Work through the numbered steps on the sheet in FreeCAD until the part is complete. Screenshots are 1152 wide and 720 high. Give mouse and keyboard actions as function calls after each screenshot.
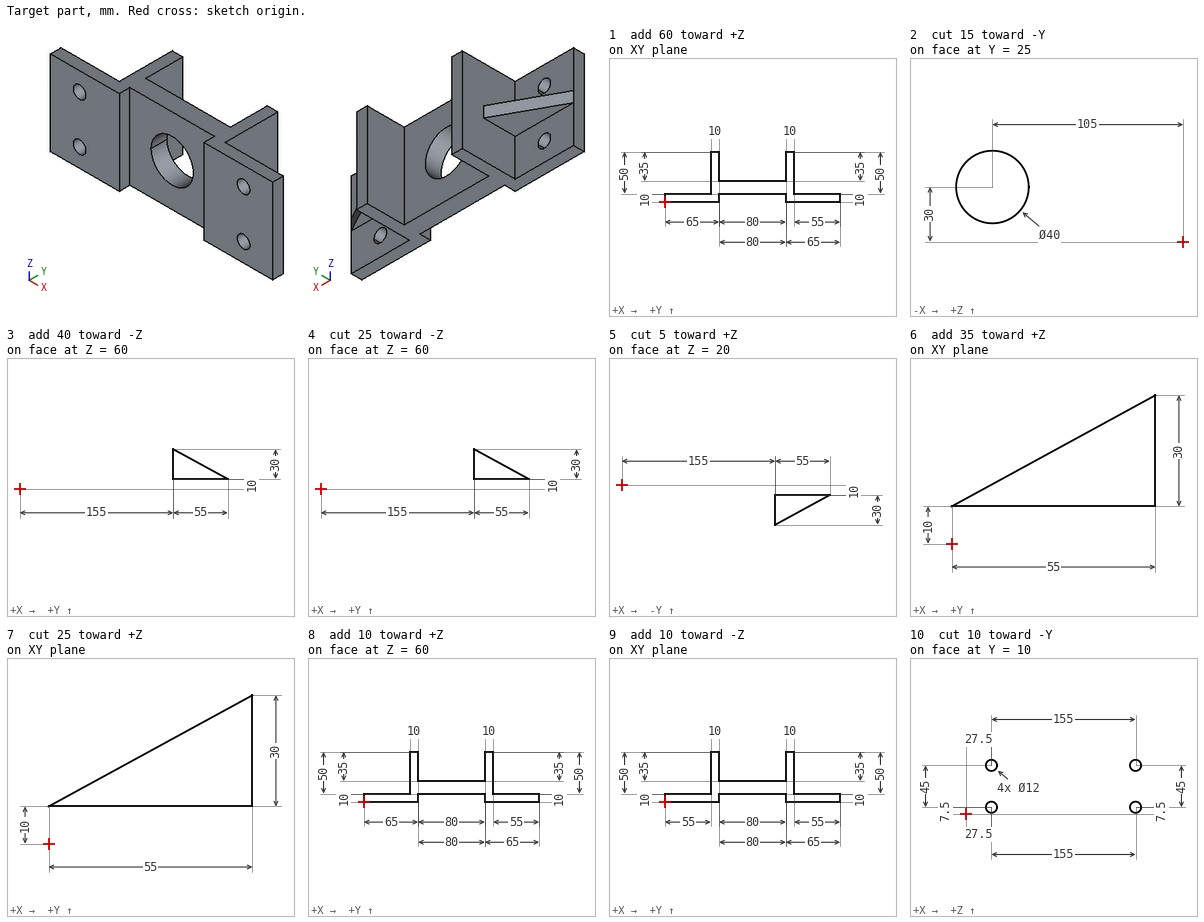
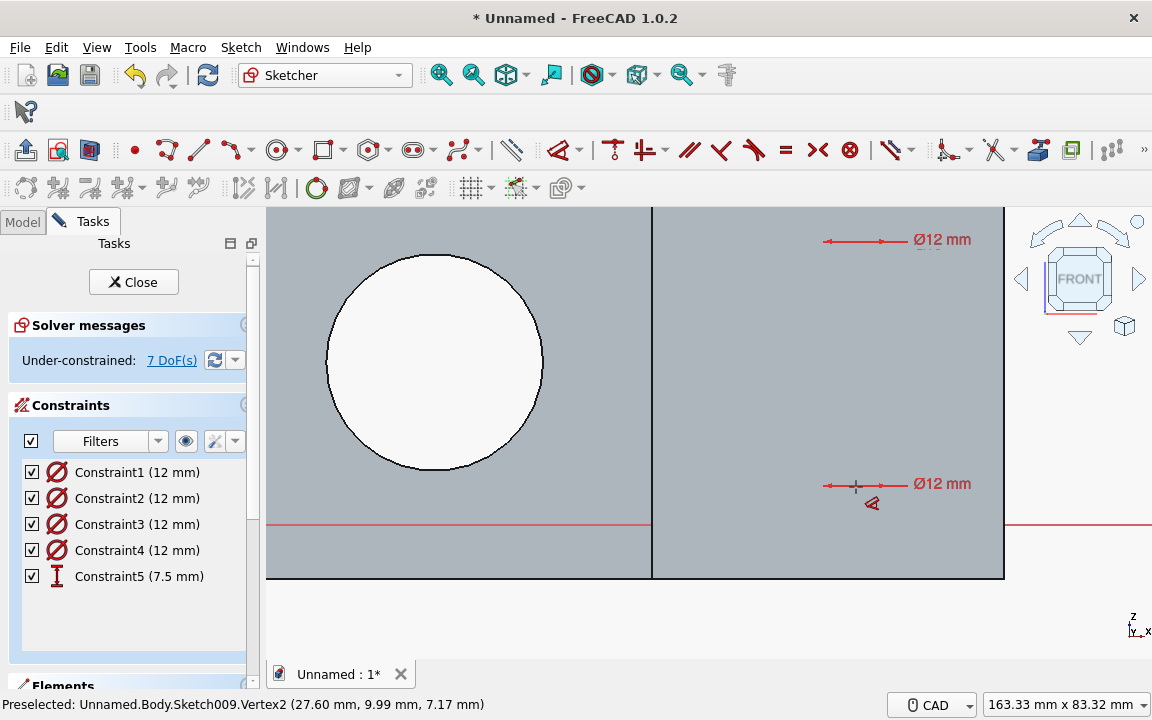
click(856, 486)
click(914, 506)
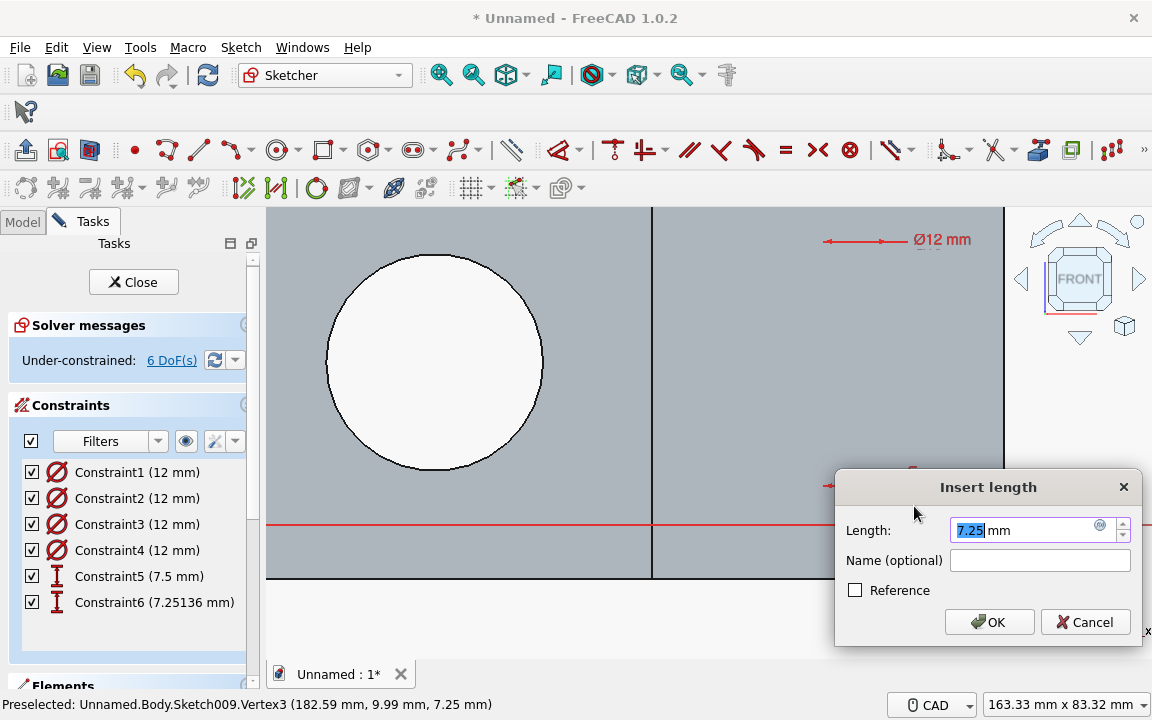
text(7.5)
key(Return)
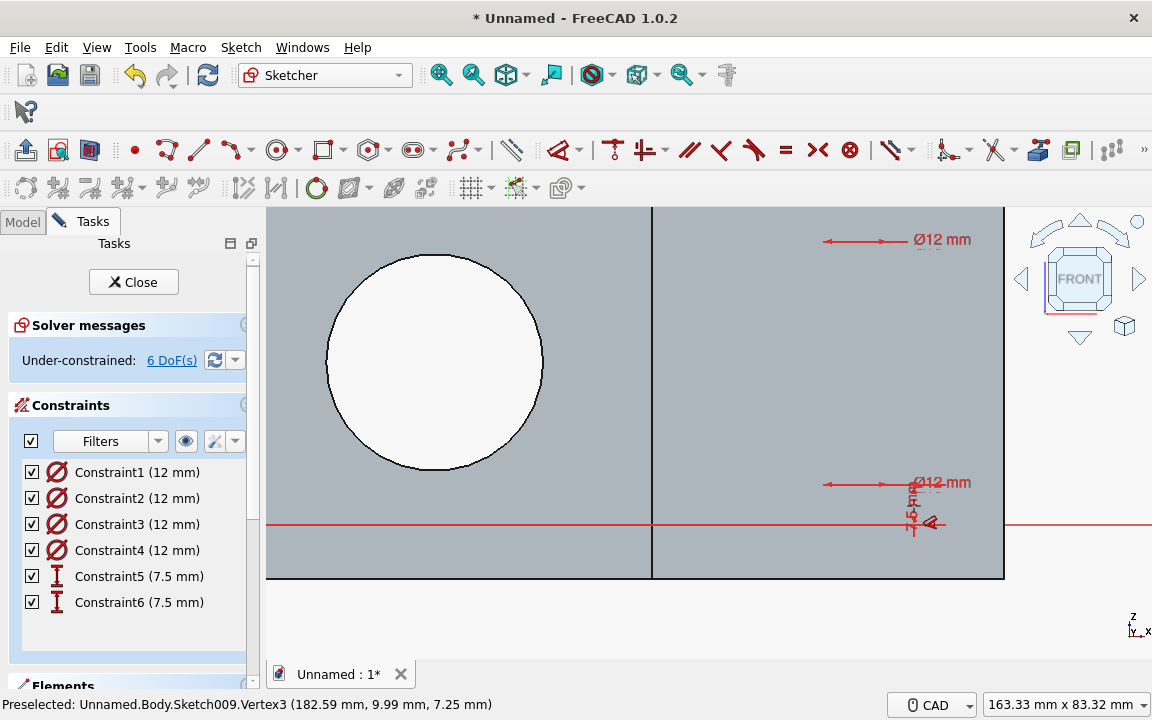
scroll(856, 487, down, 4)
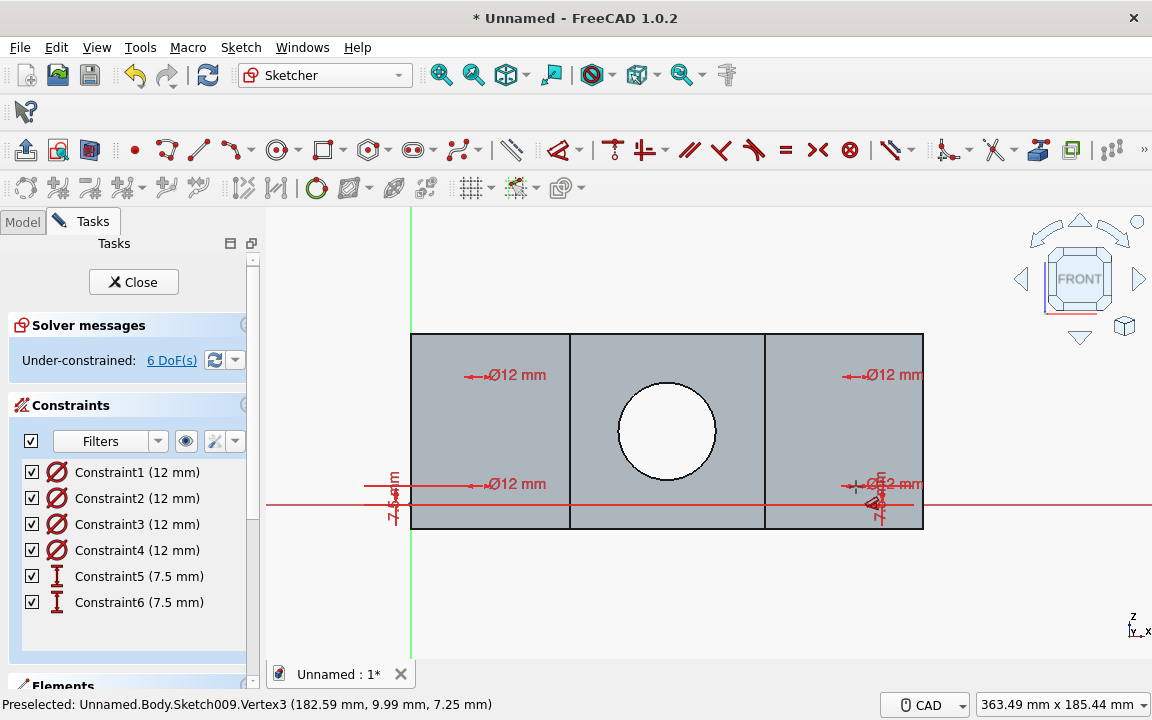
click(478, 377)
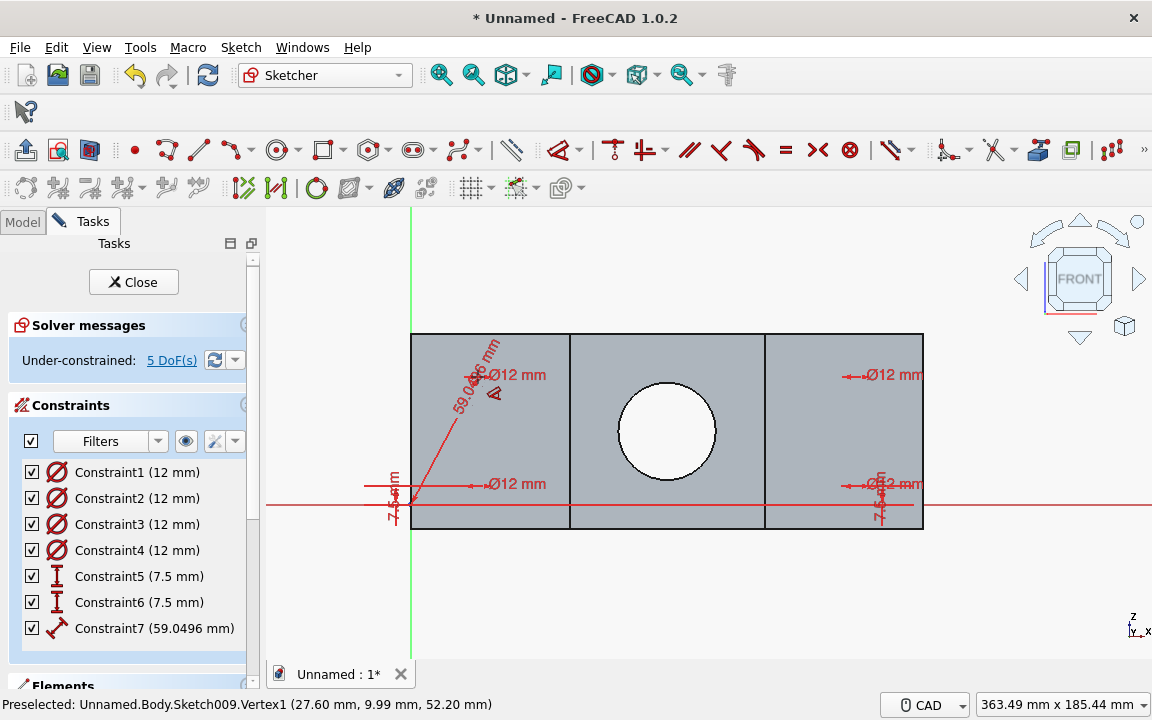
click(478, 486)
click(444, 432)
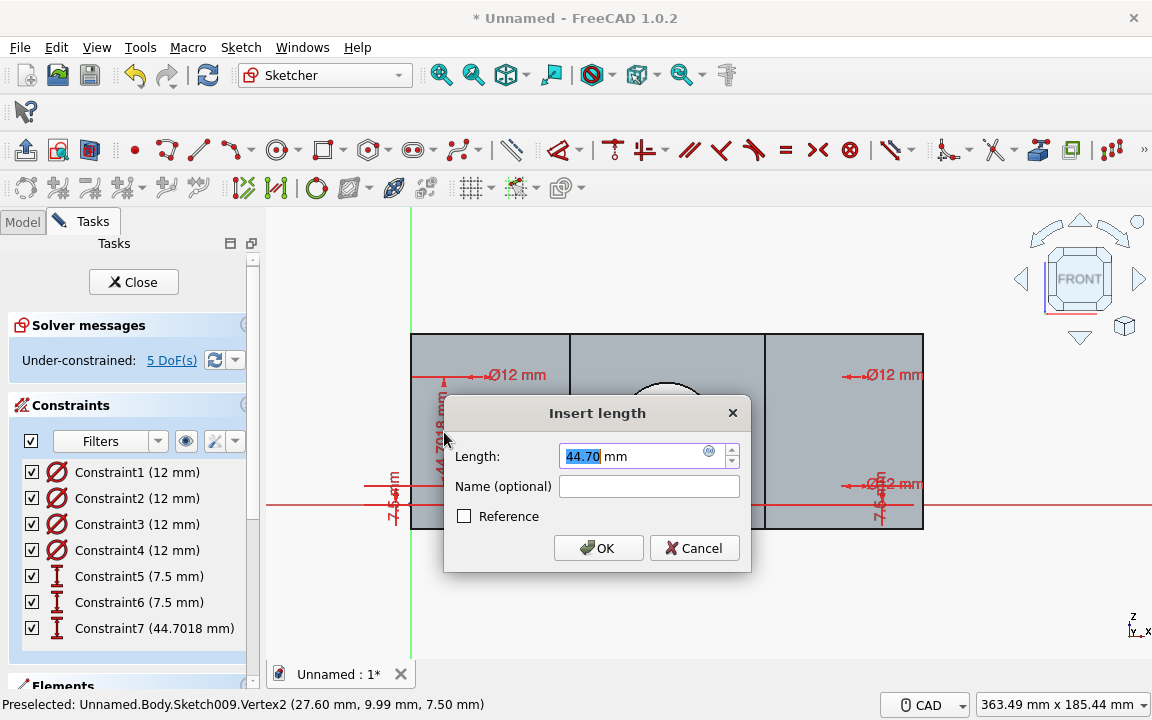
text(45)
key(Return)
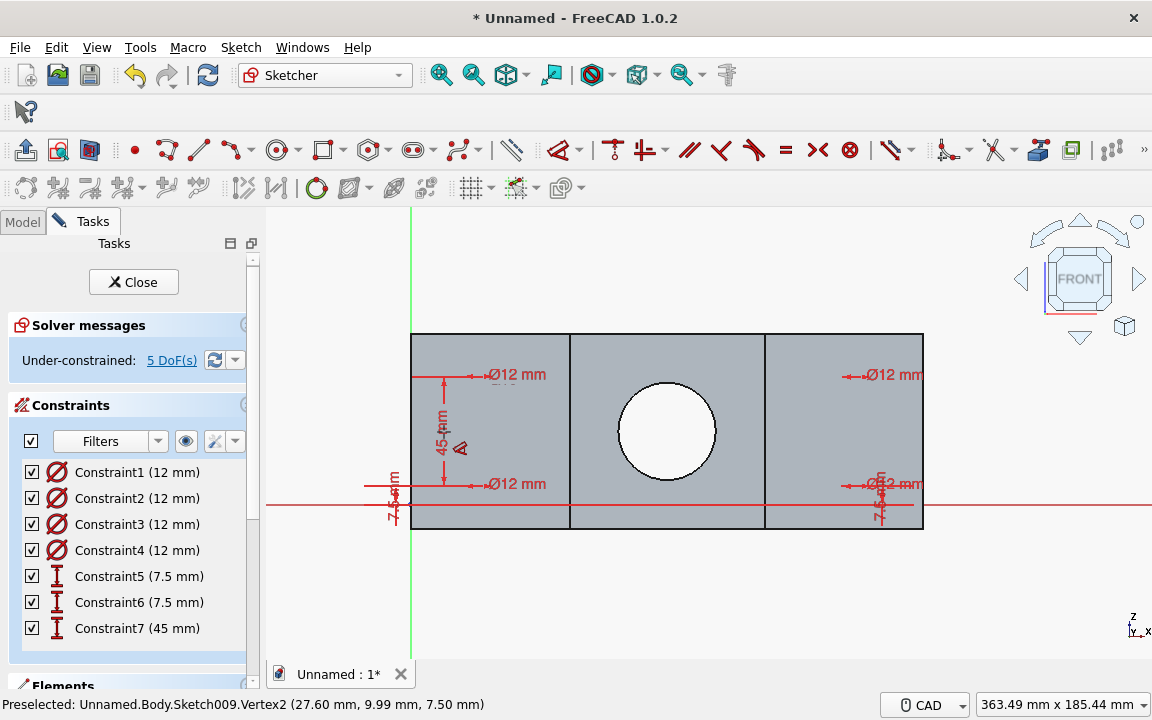
click(856, 486)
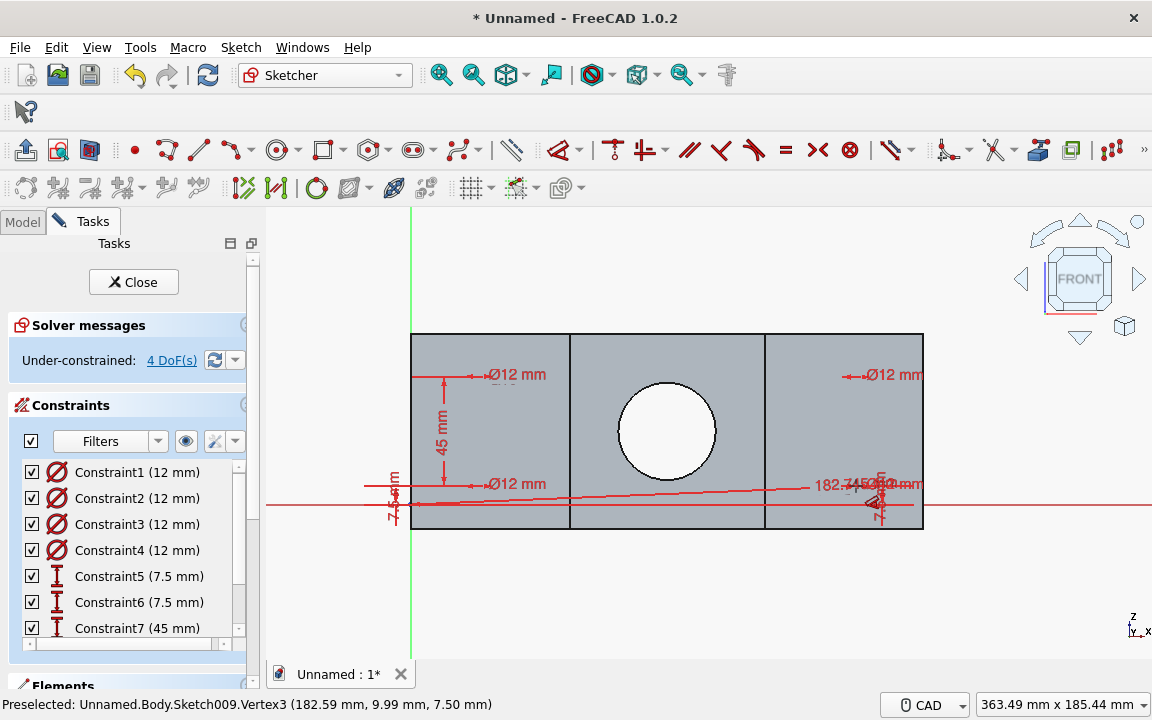
click(856, 377)
click(890, 432)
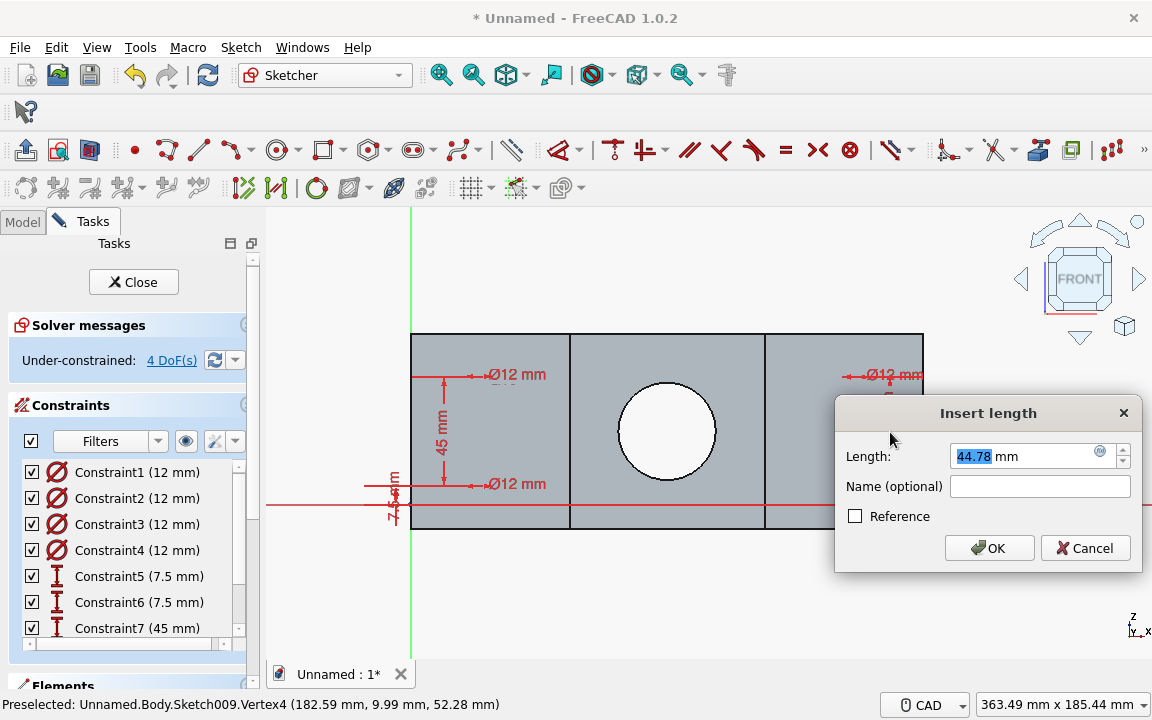
text(45)
key(Return)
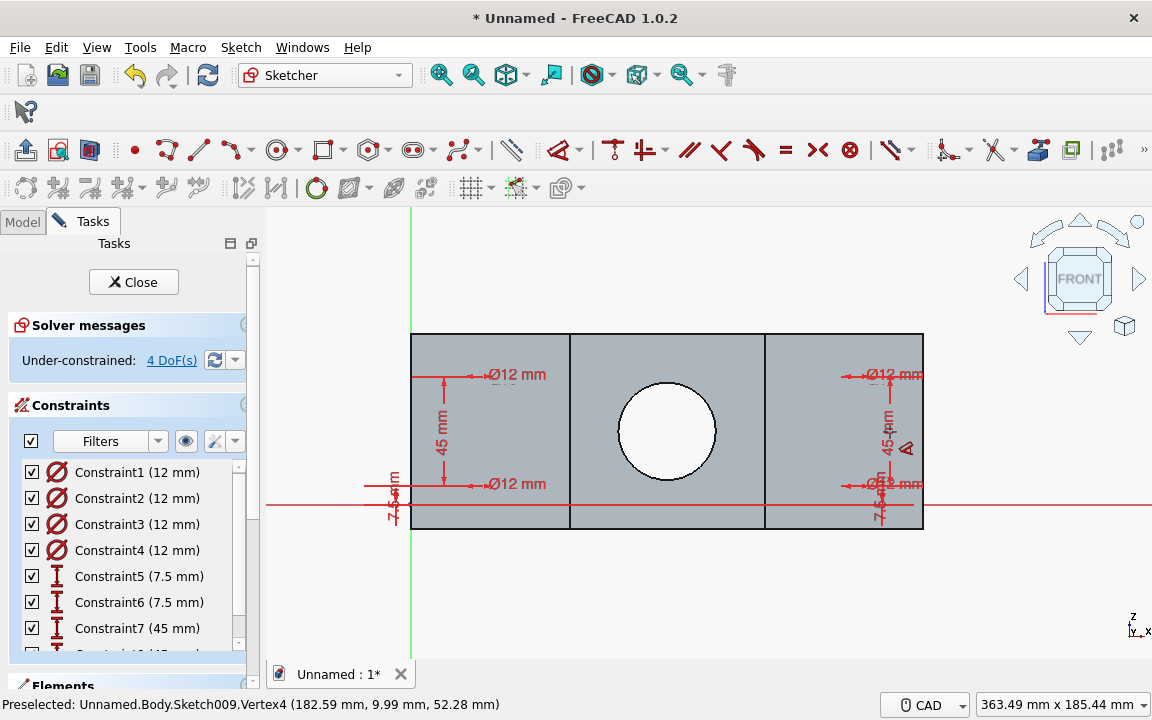
click(478, 377)
click(445, 539)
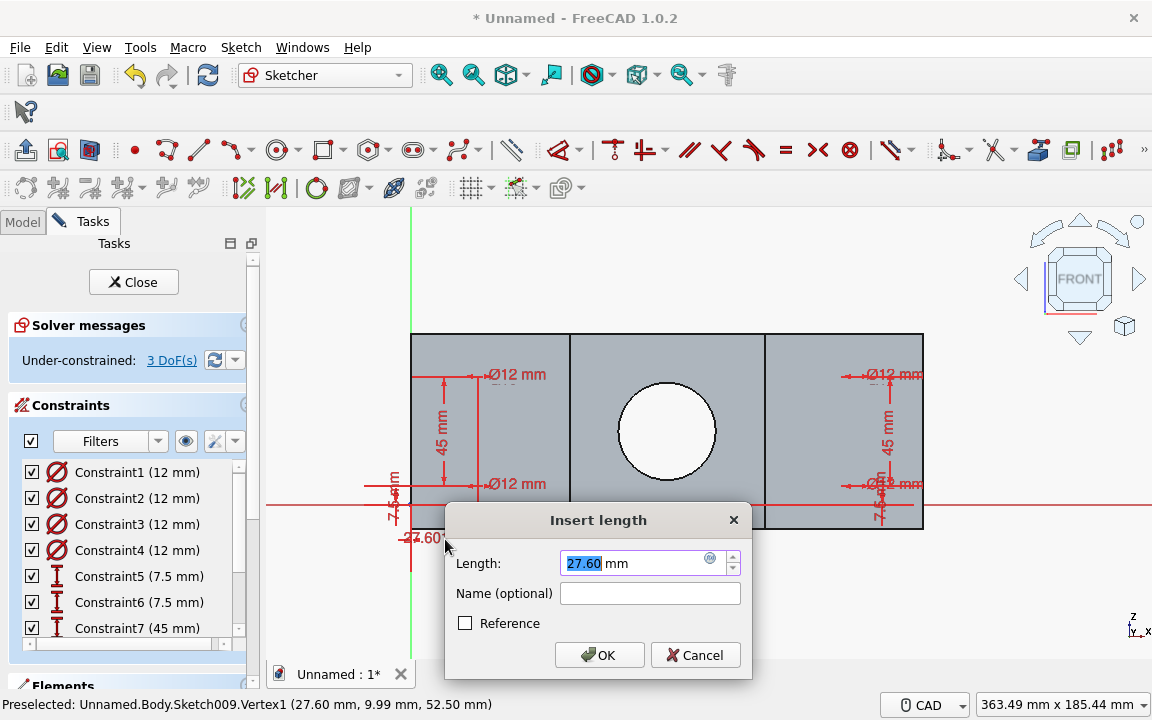
text(27.5)
key(Return)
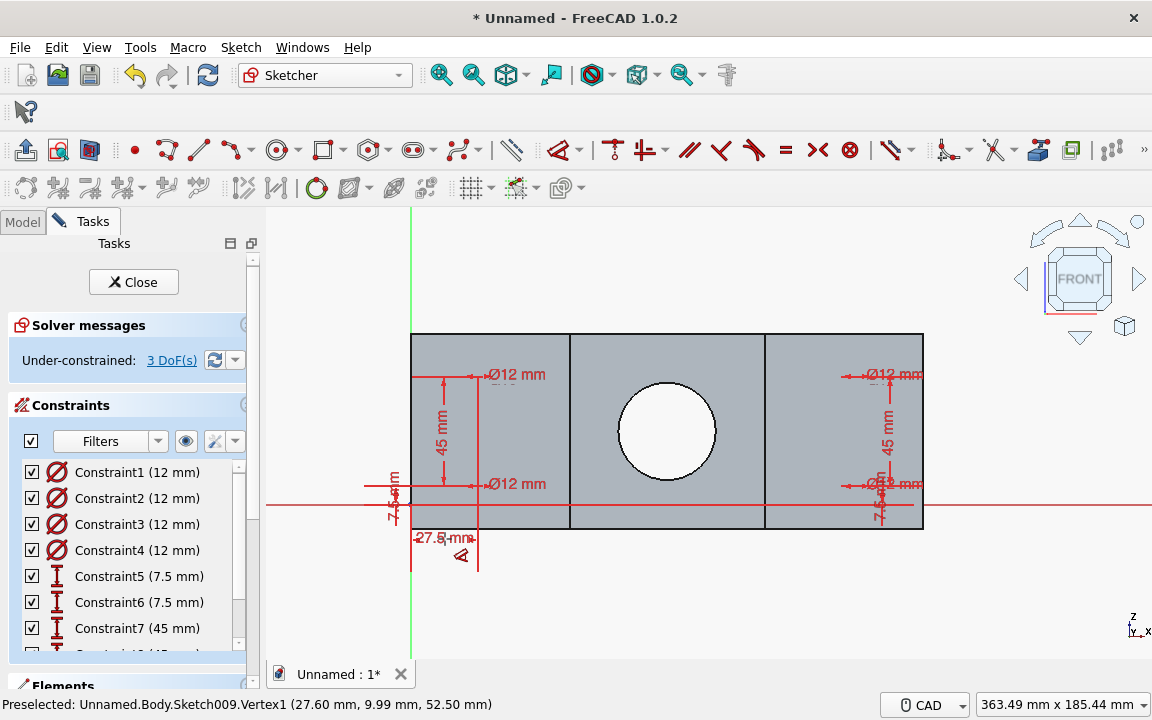
click(478, 486)
click(445, 452)